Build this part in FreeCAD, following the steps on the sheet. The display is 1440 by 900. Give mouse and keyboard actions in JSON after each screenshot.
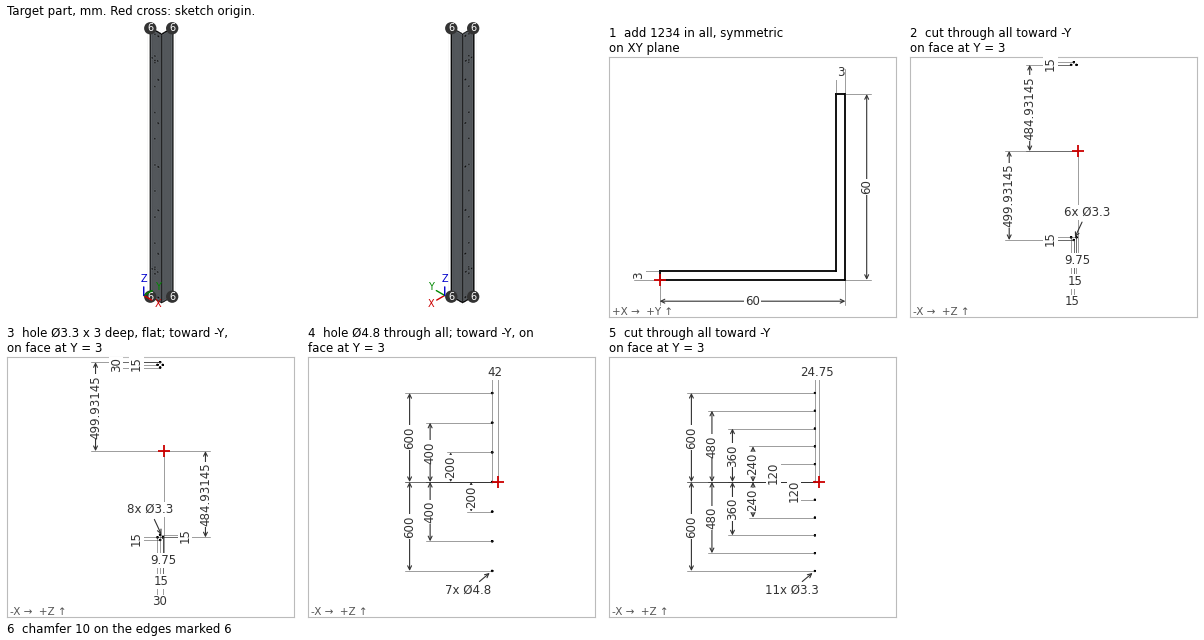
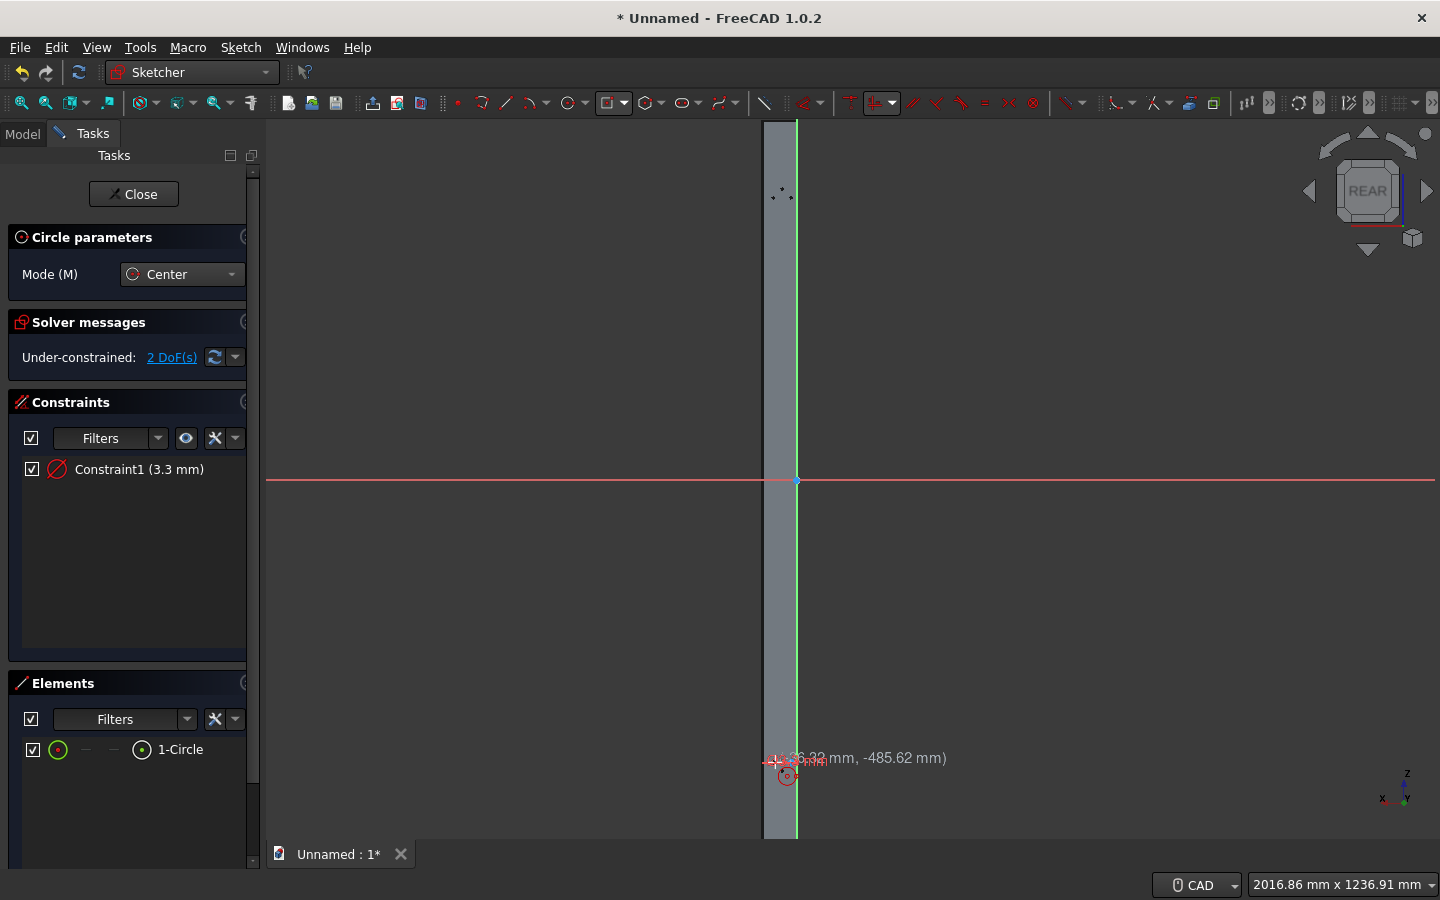
{"action": "left_click", "coordinate": [773, 762]}
{"action": "mouse_move", "coordinate": [774, 762]}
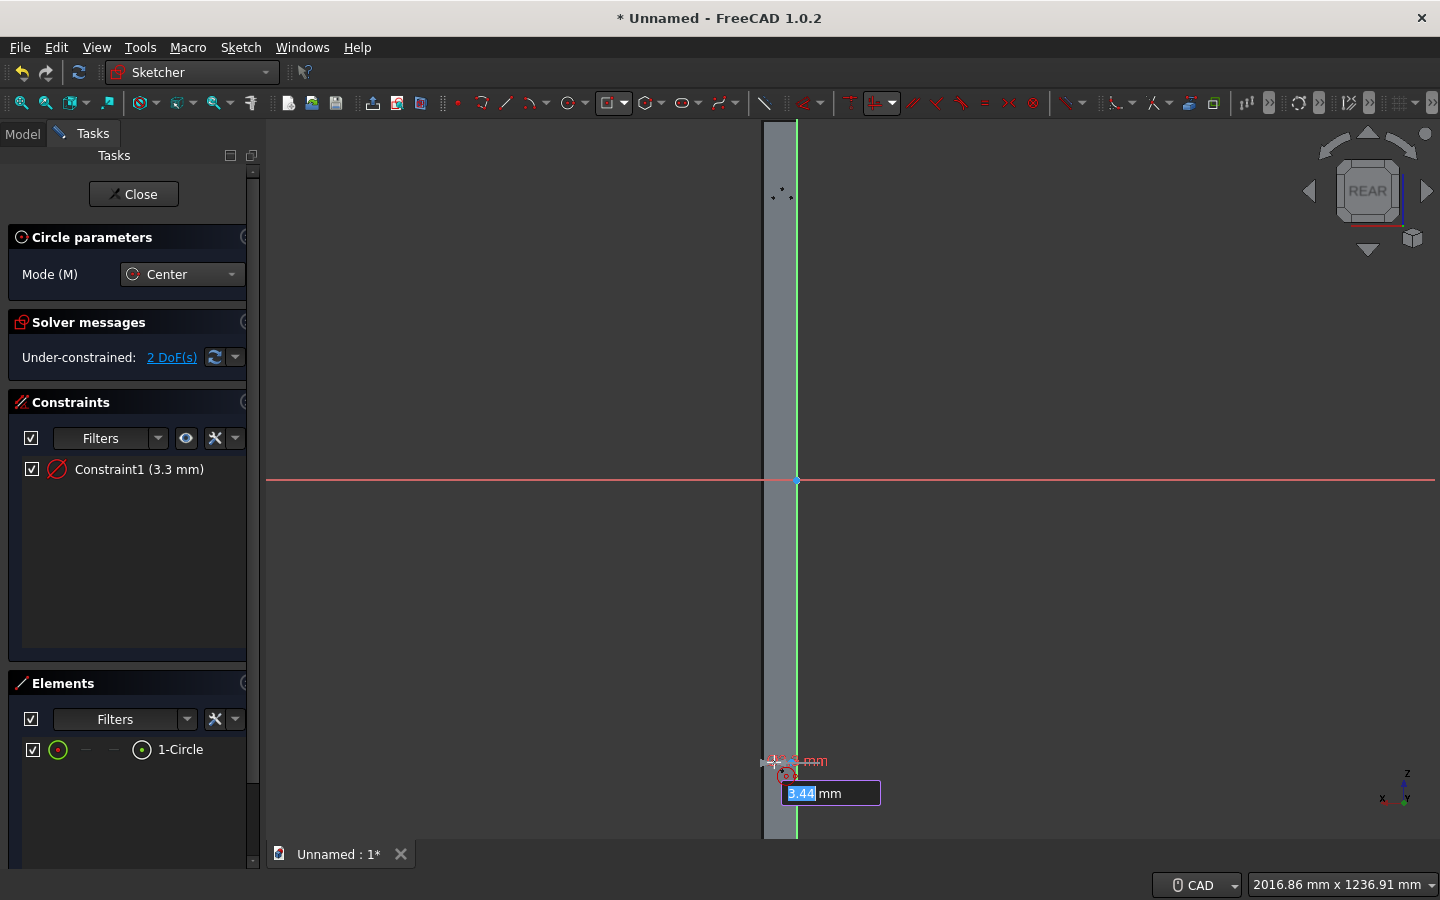
{"action": "type", "text": "3.3"}
{"action": "key", "text": "Return"}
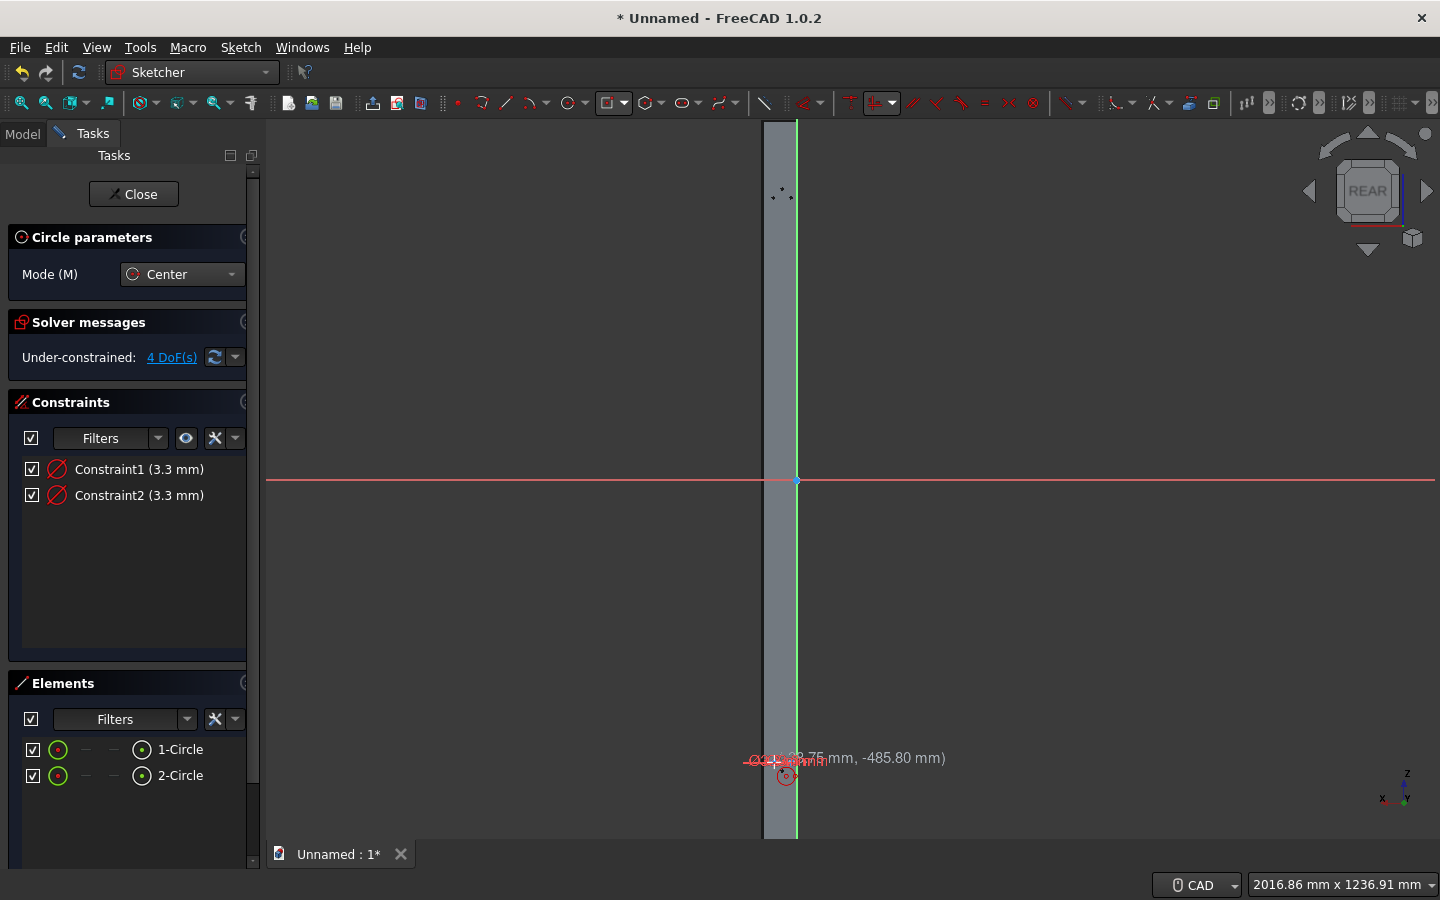
{"action": "scroll", "coordinate": [782, 754], "scroll_direction": "up", "scroll_amount": 16}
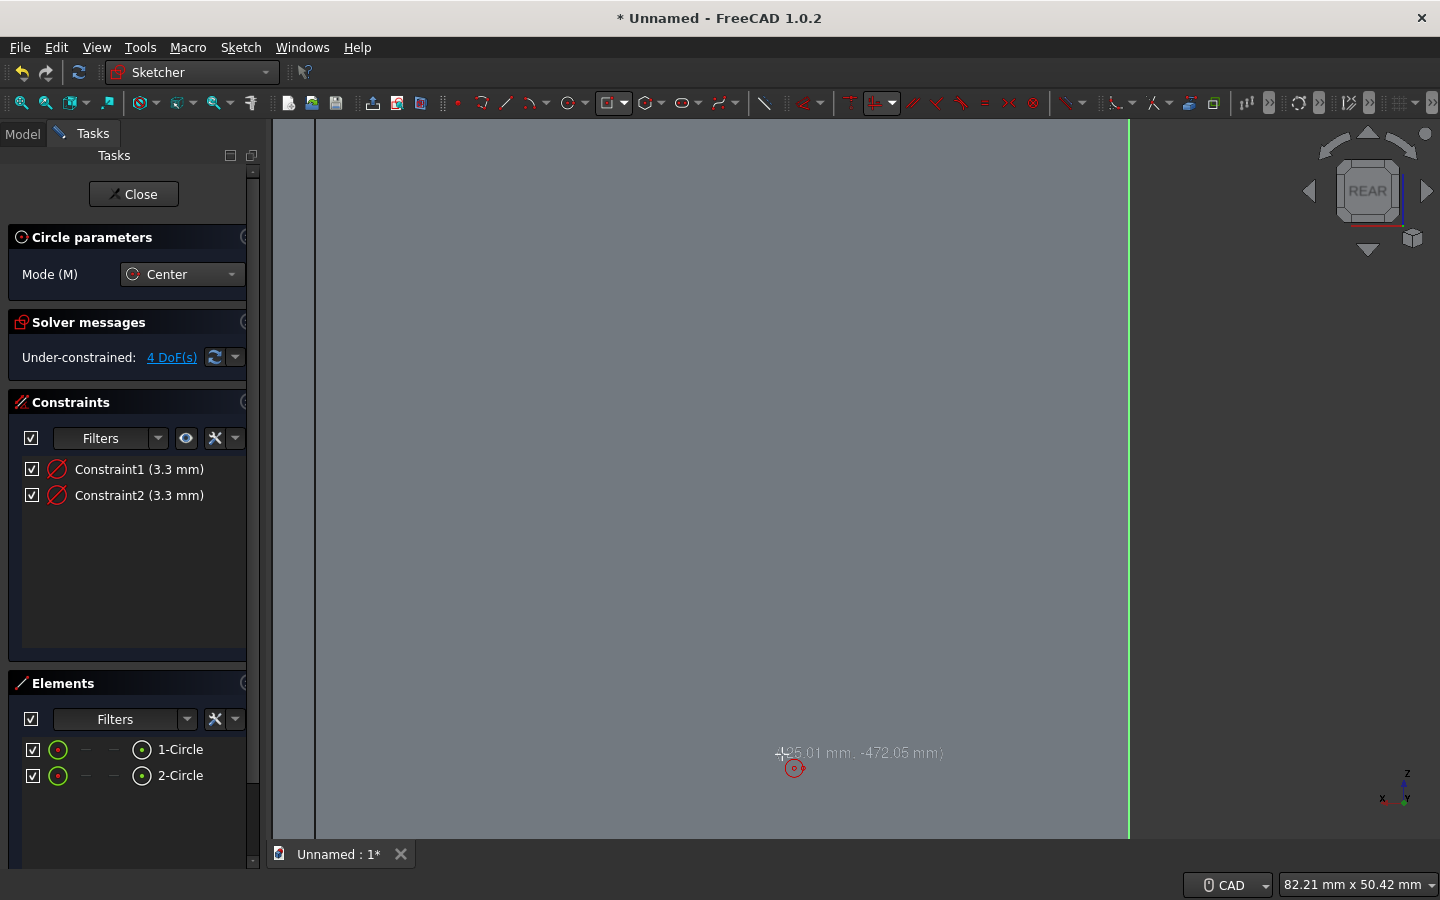
{"action": "scroll", "coordinate": [782, 754], "scroll_direction": "down", "scroll_amount": 16}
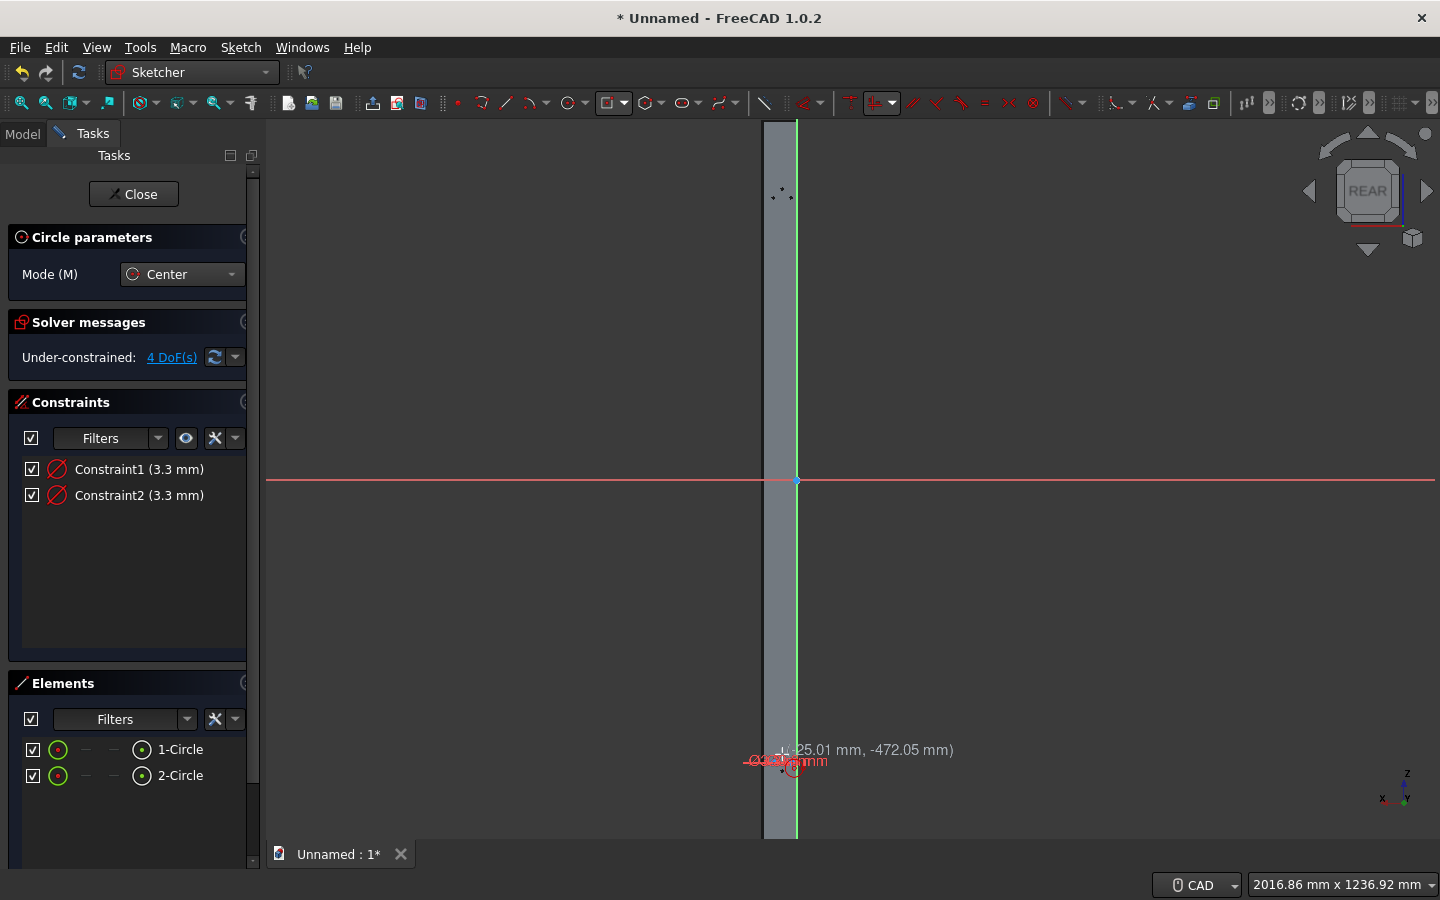
{"action": "scroll", "coordinate": [782, 754], "scroll_direction": "up", "scroll_amount": 2}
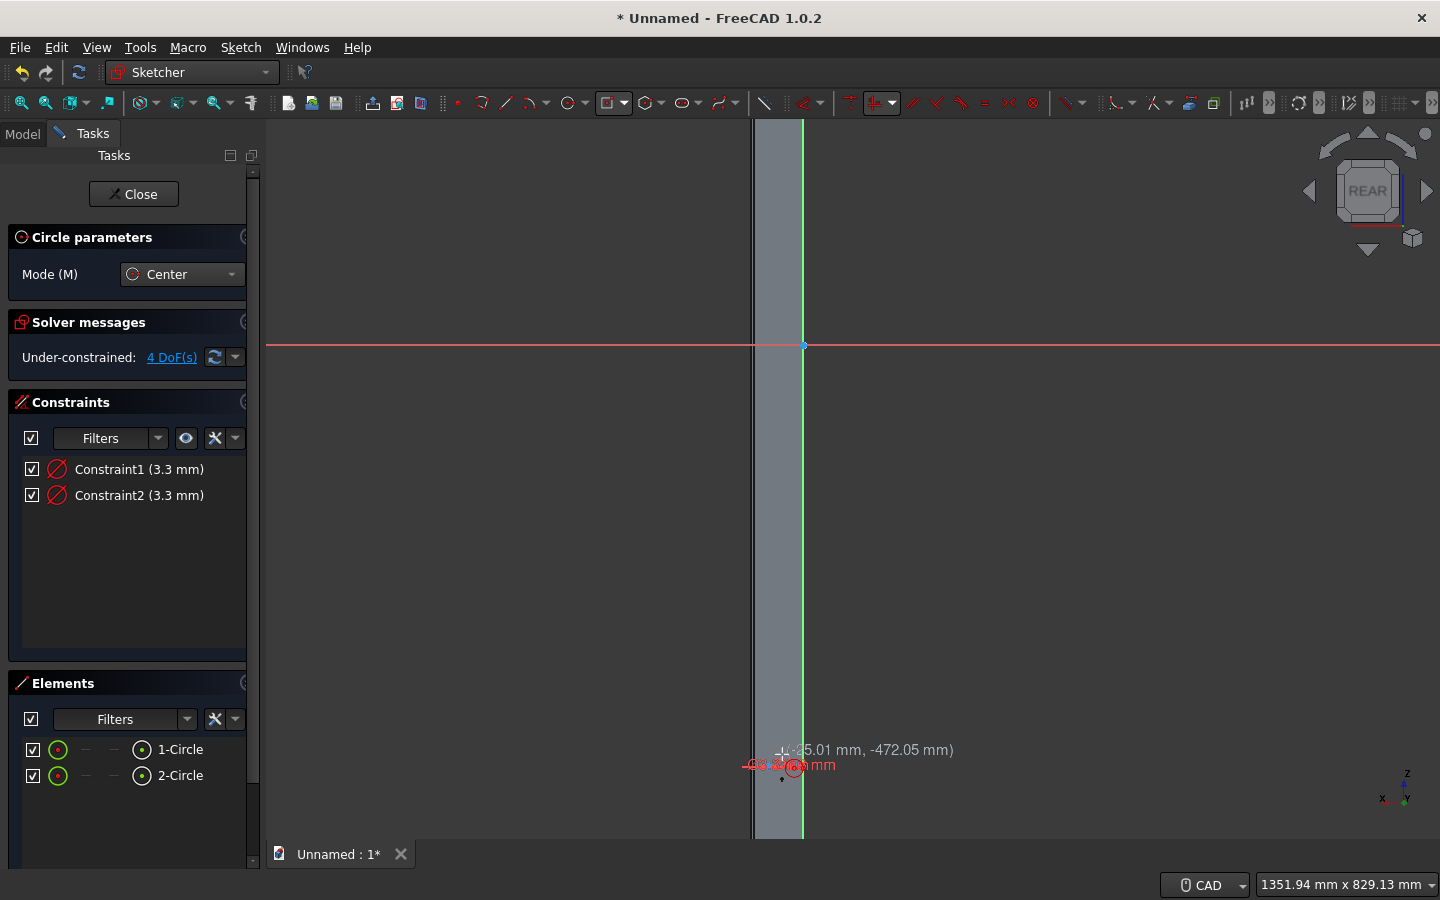
{"action": "left_click", "coordinate": [782, 753]}
{"action": "mouse_move", "coordinate": [783, 752]}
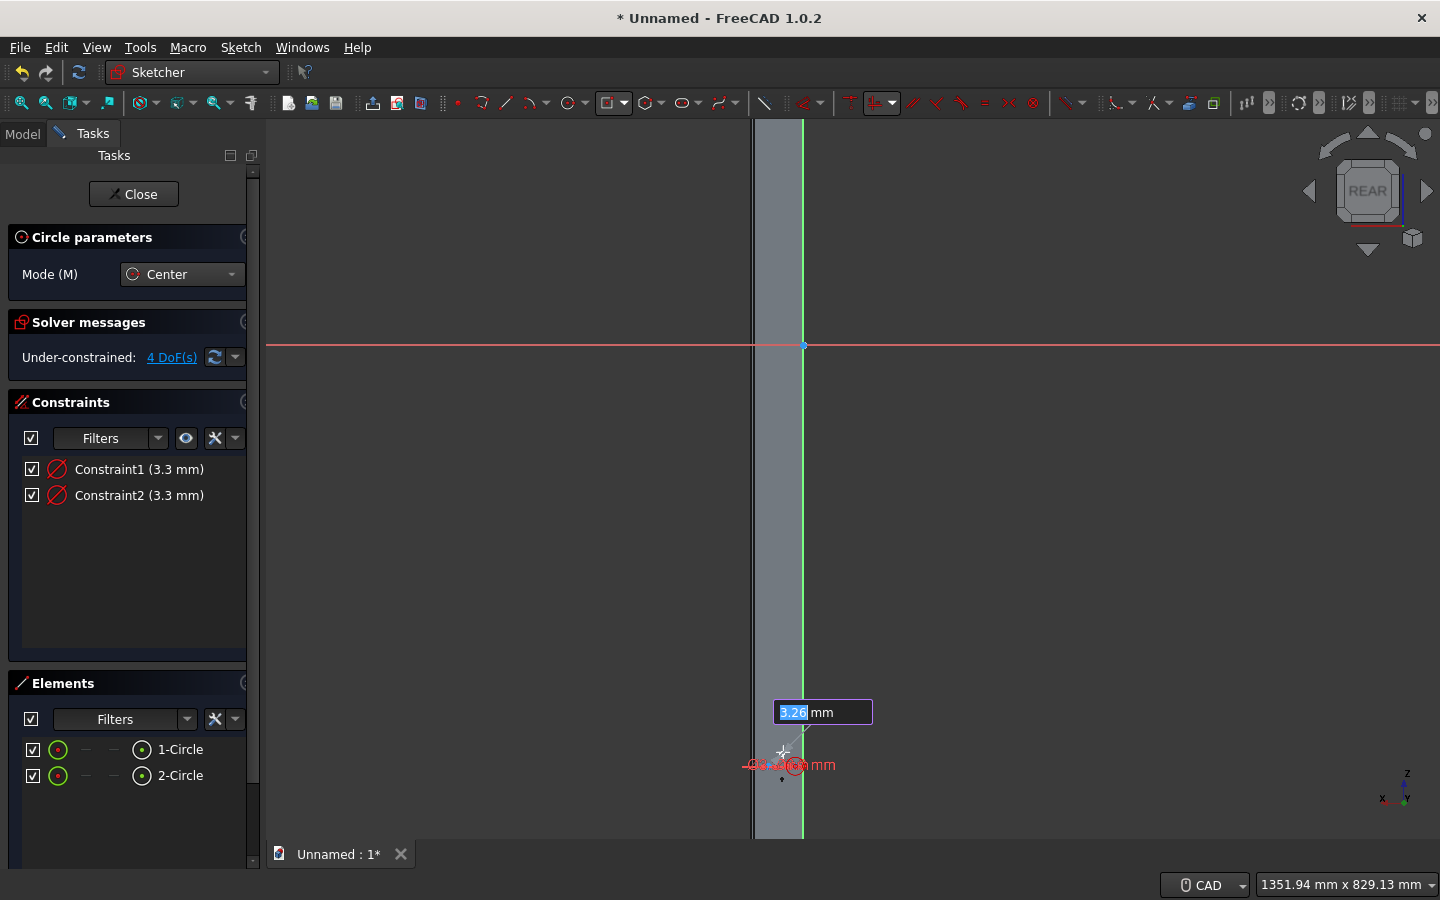
{"action": "type", "text": "3.3"}
{"action": "key", "text": "Return"}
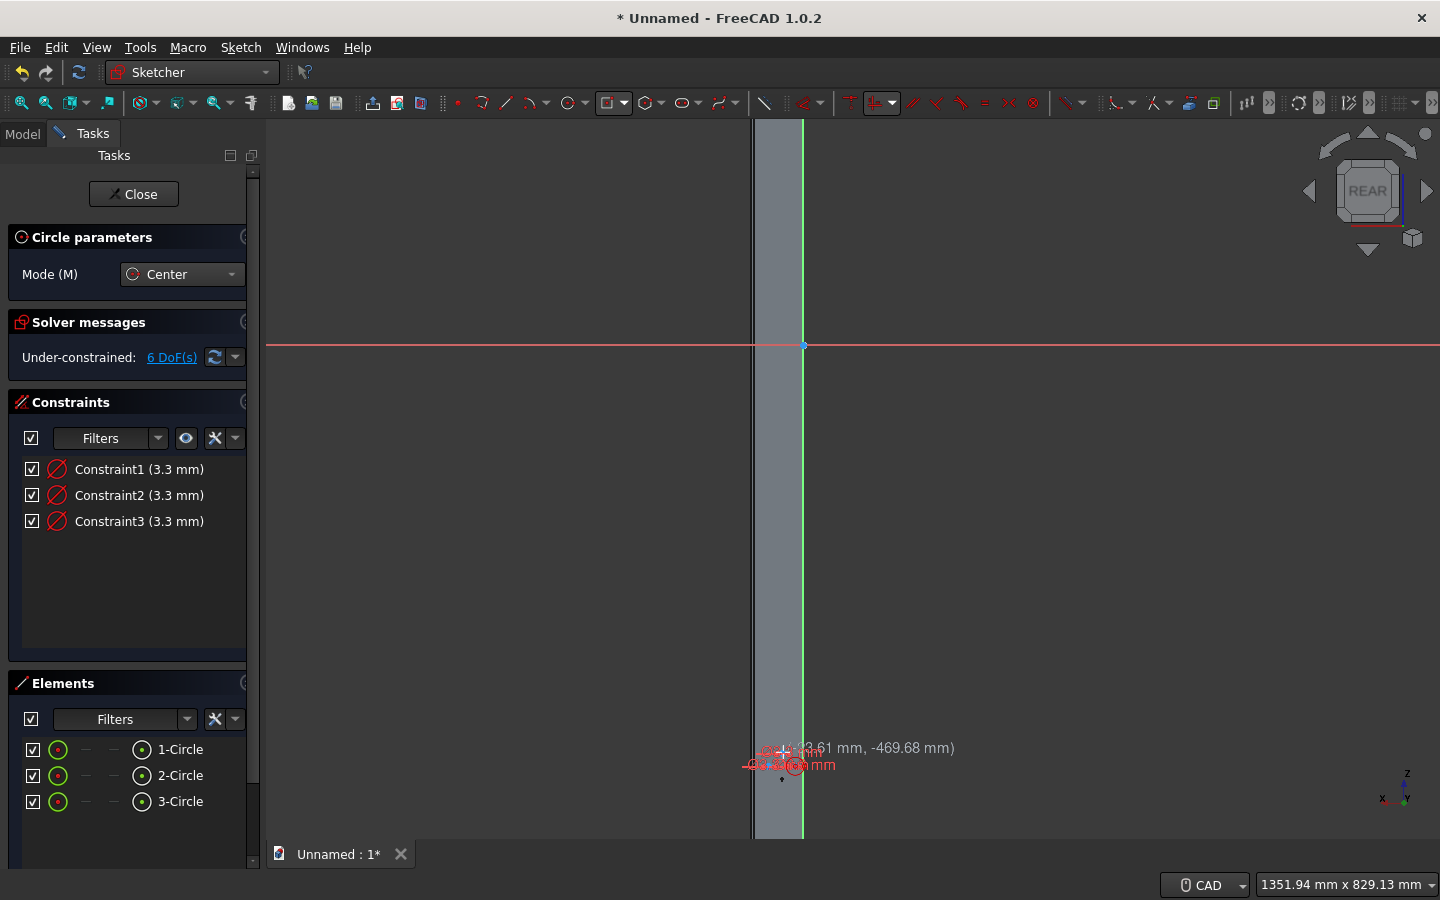
{"action": "scroll", "coordinate": [782, 779], "scroll_direction": "up", "scroll_amount": 14}